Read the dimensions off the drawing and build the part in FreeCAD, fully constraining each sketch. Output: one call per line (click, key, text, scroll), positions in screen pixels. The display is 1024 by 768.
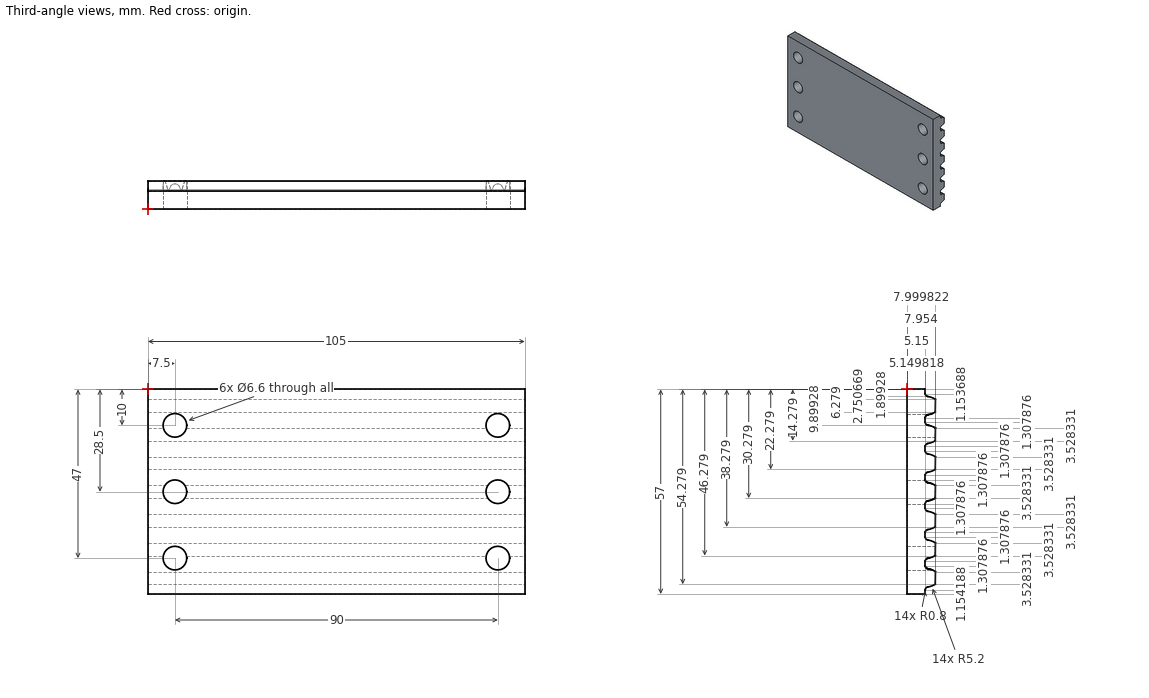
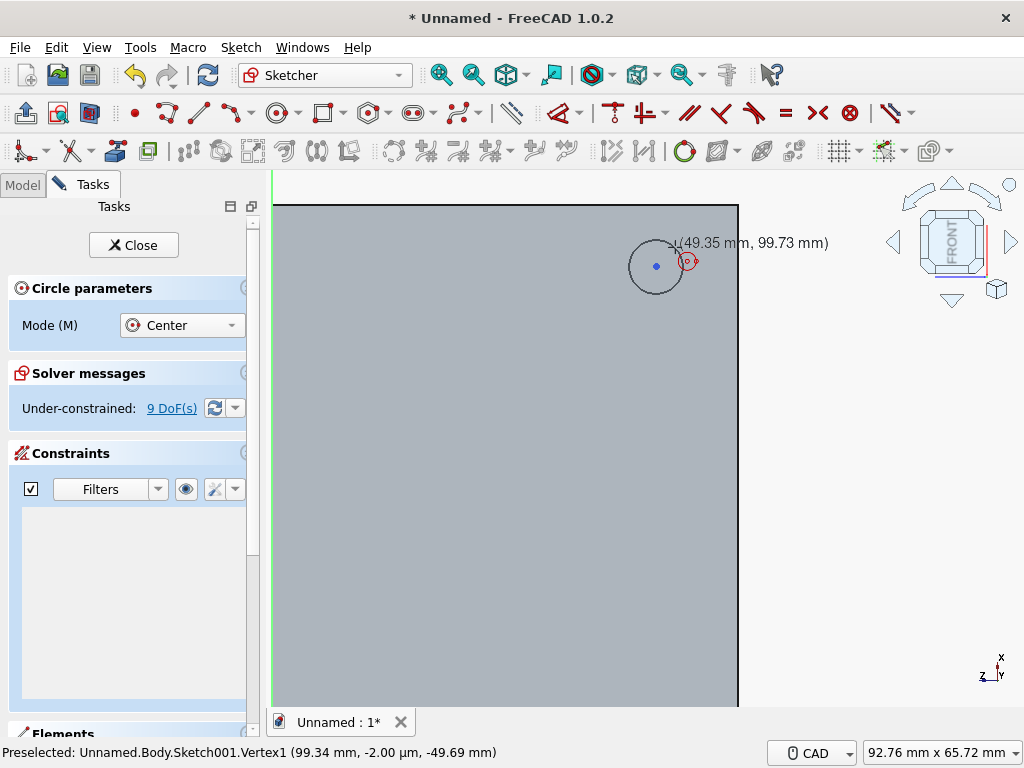
click(353, 266)
click(373, 247)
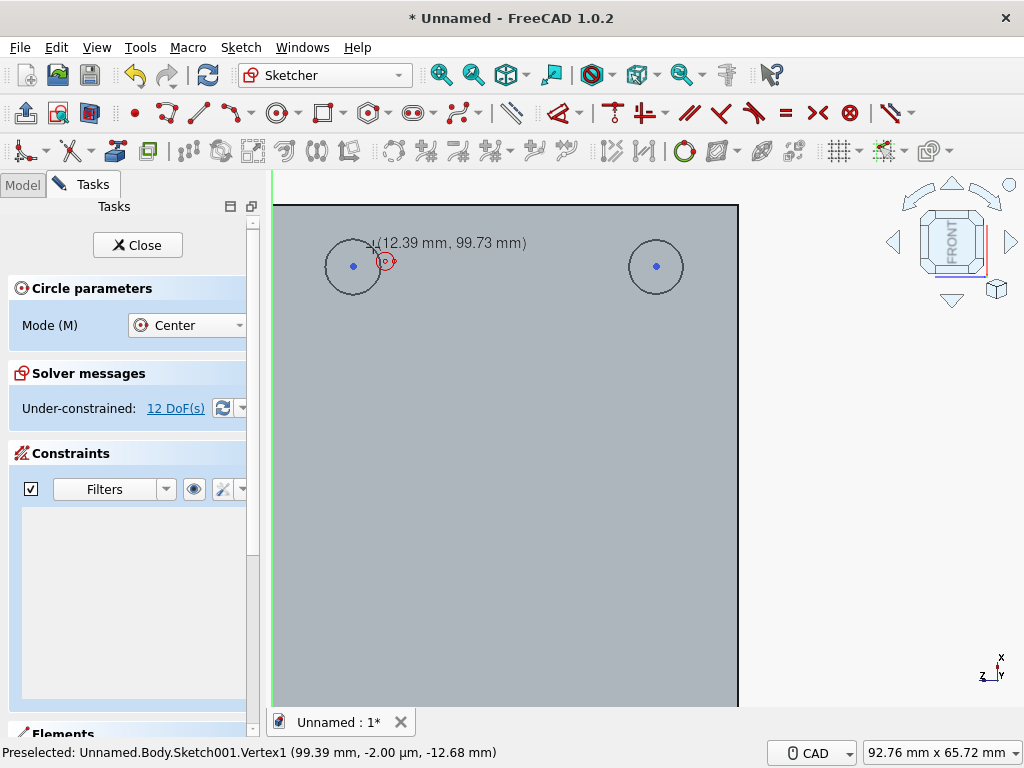
click(505, 266)
click(524, 247)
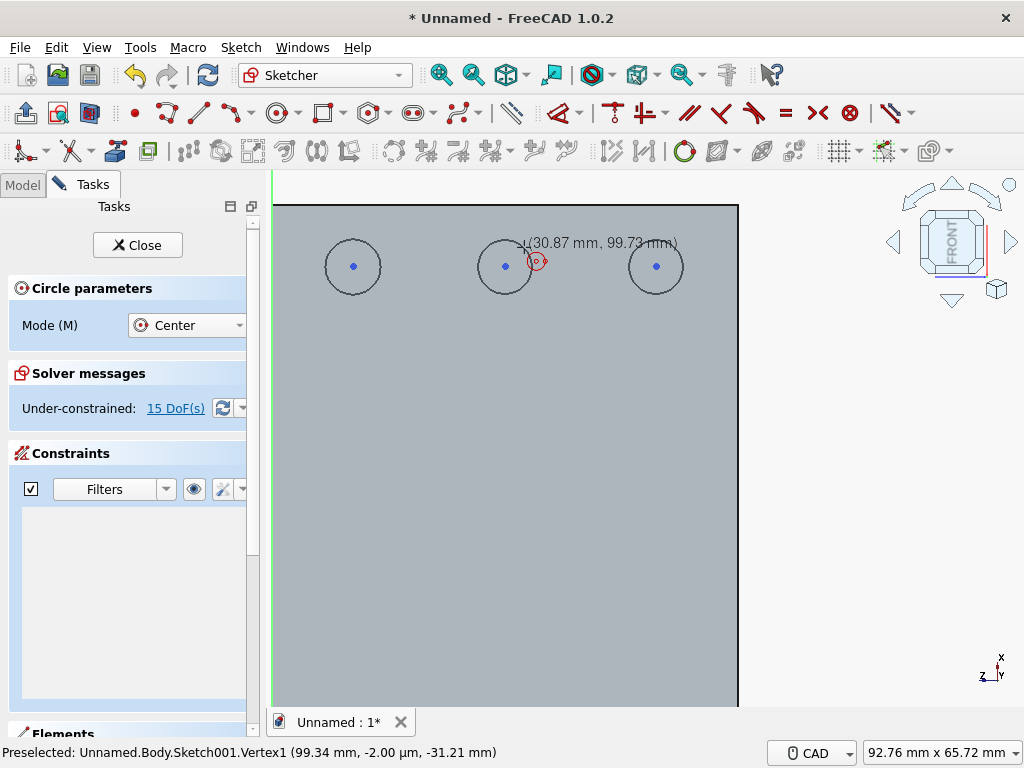
scroll(657, 265, down, 4)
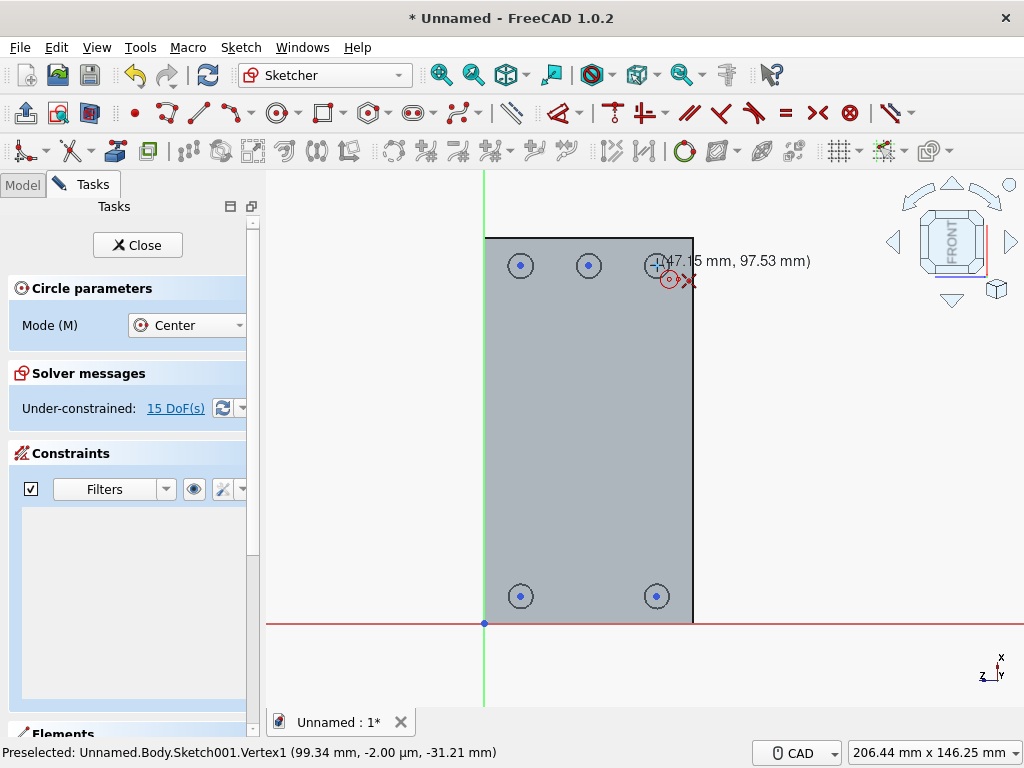
scroll(589, 596, up, 4)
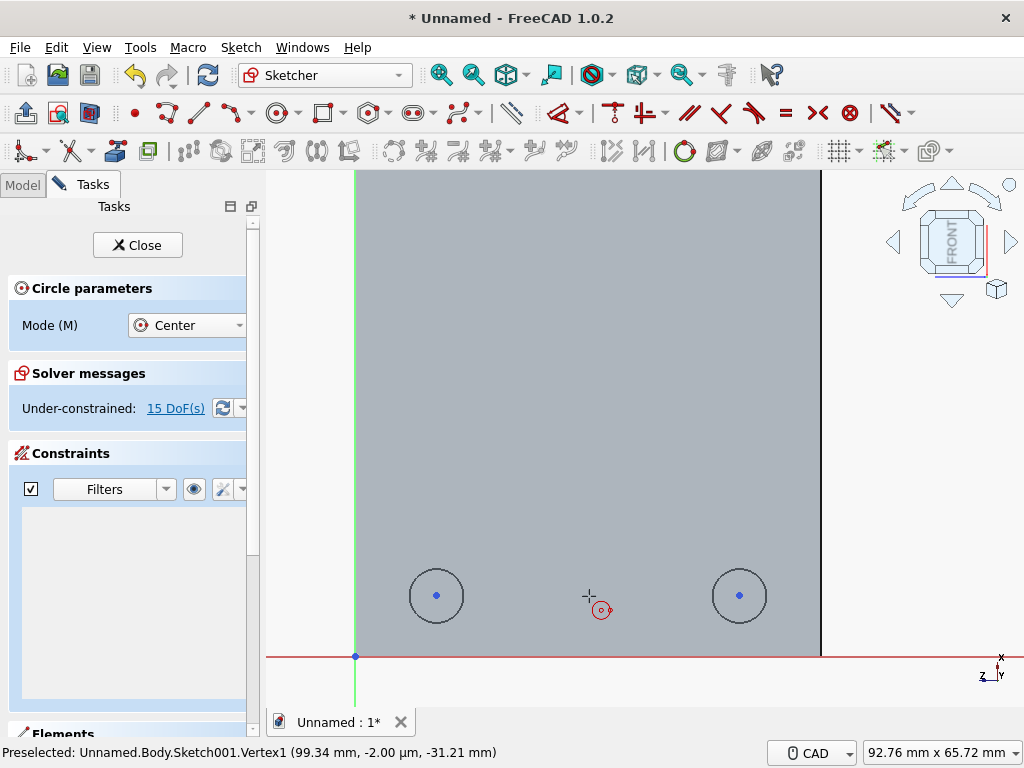
click(588, 595)
click(607, 576)
key(Escape)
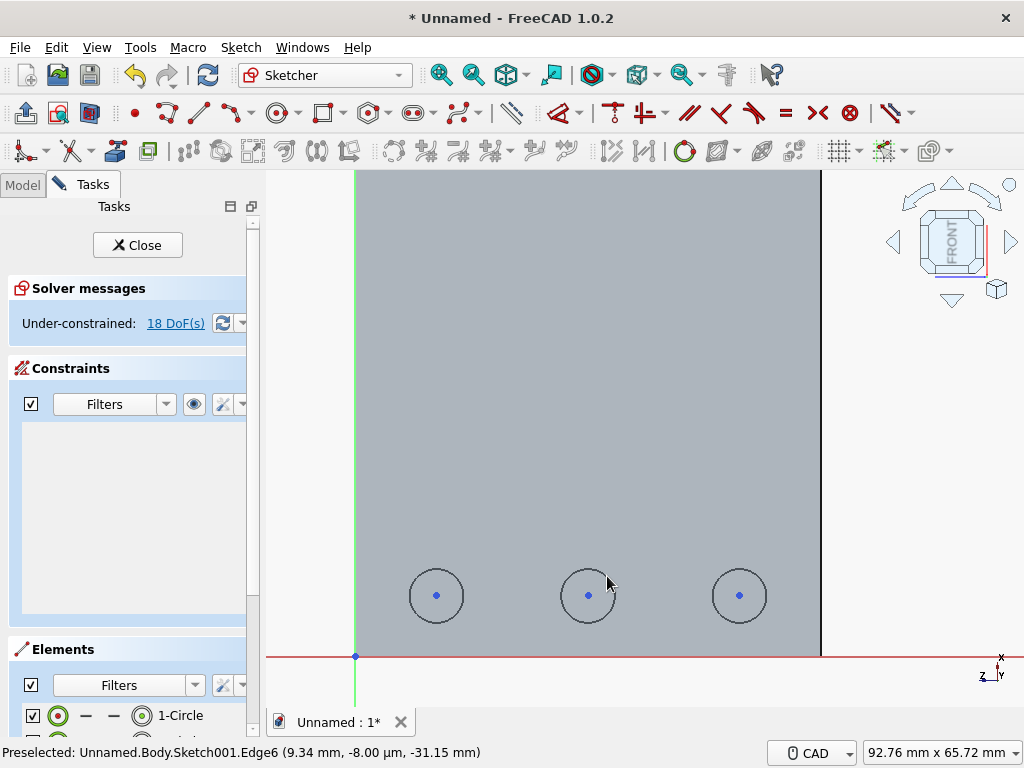
click(455, 577)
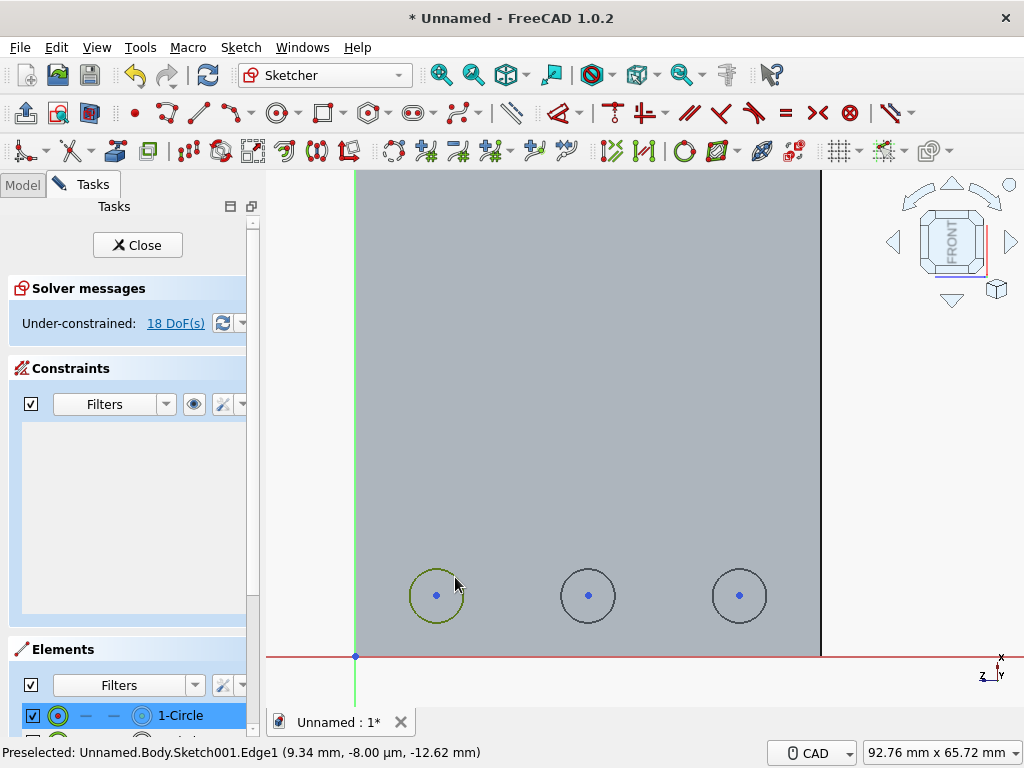
click(758, 577)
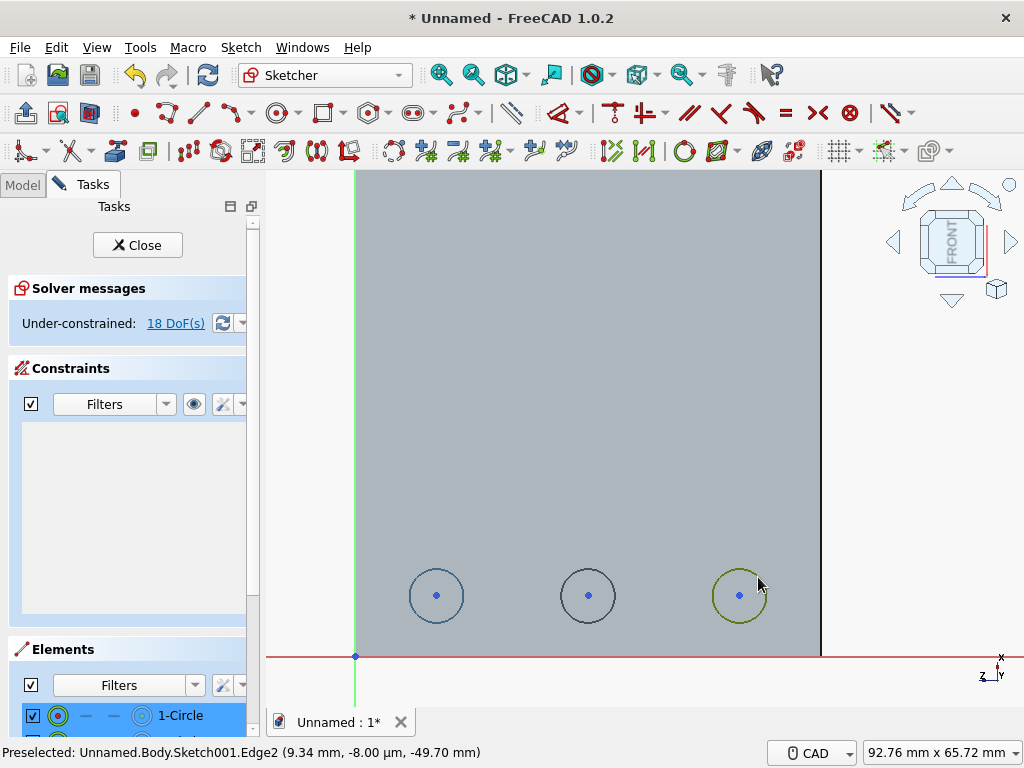
scroll(589, 597, down, 4)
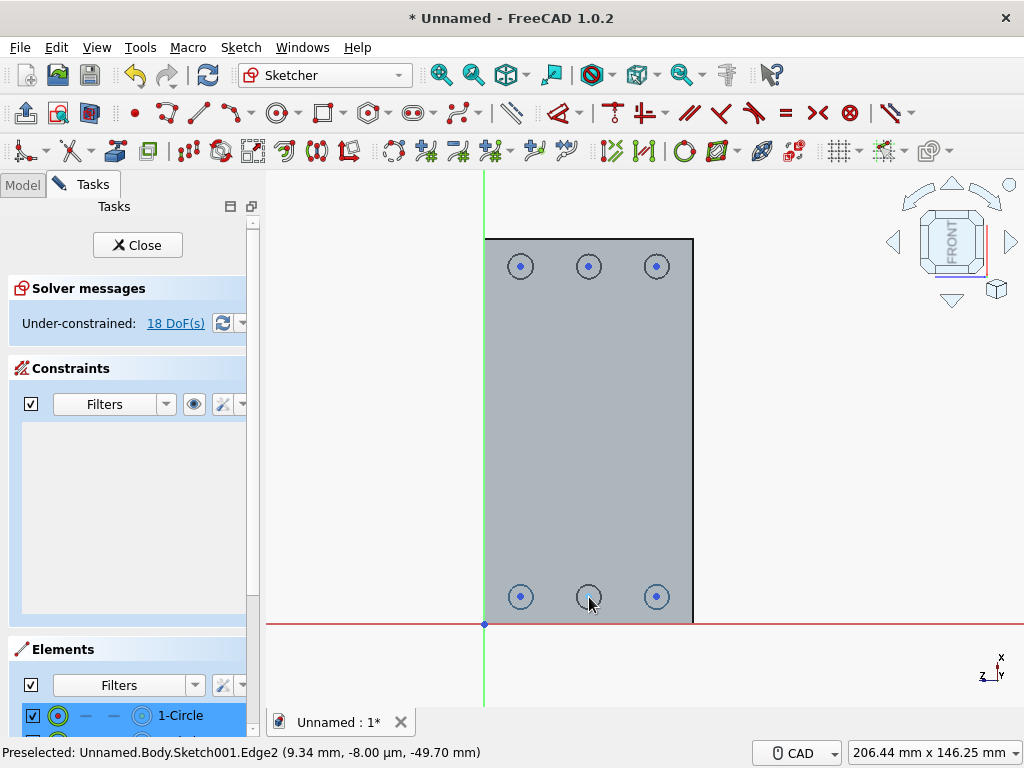
click(665, 258)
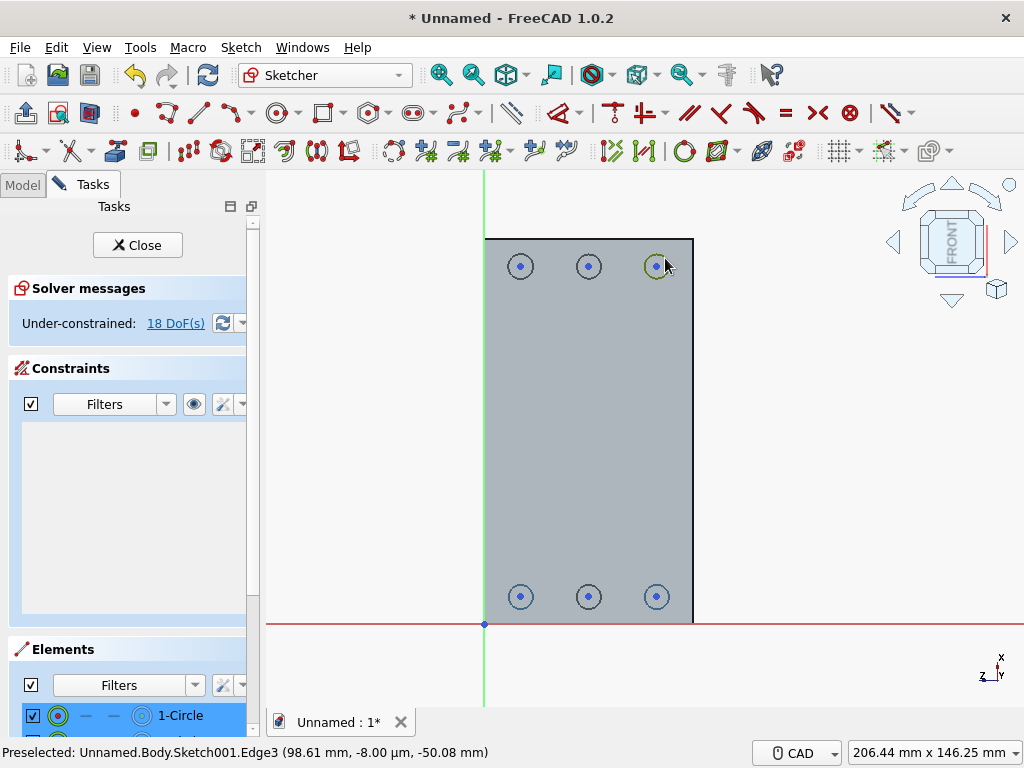
click(529, 258)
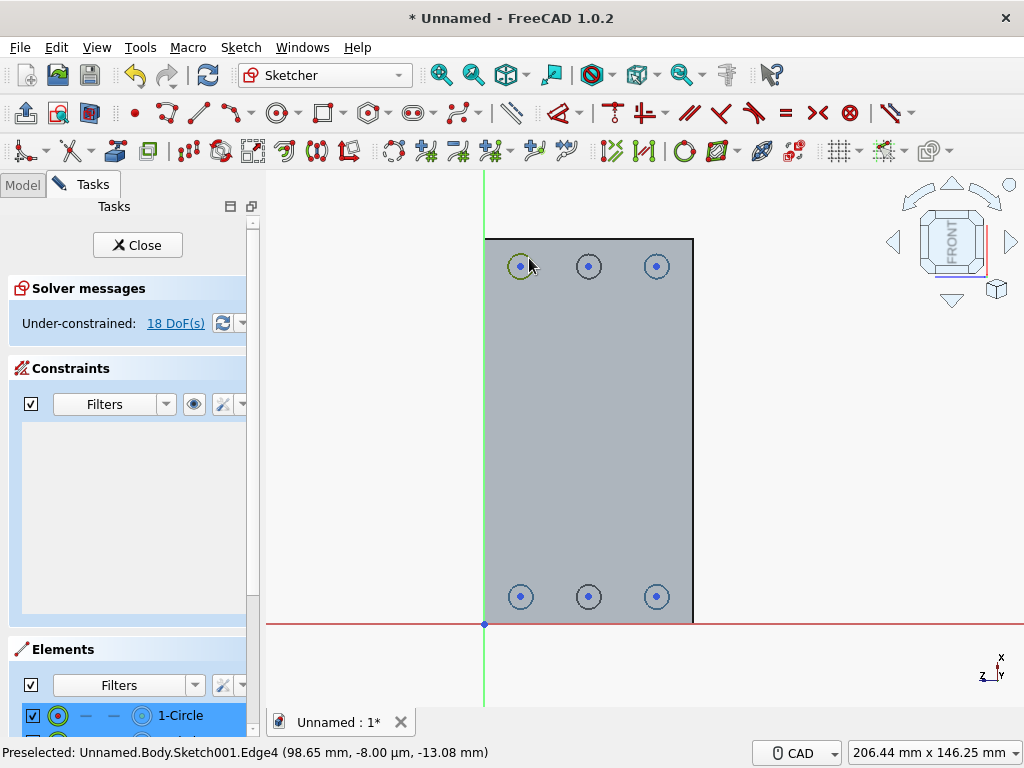
click(597, 258)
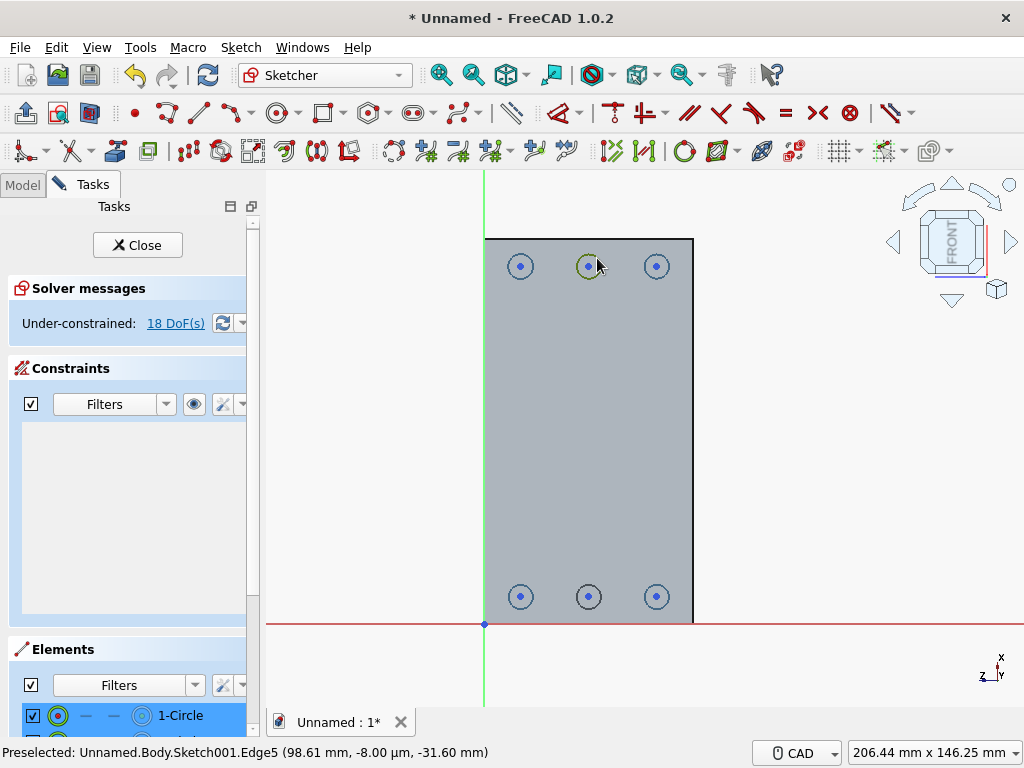
click(597, 588)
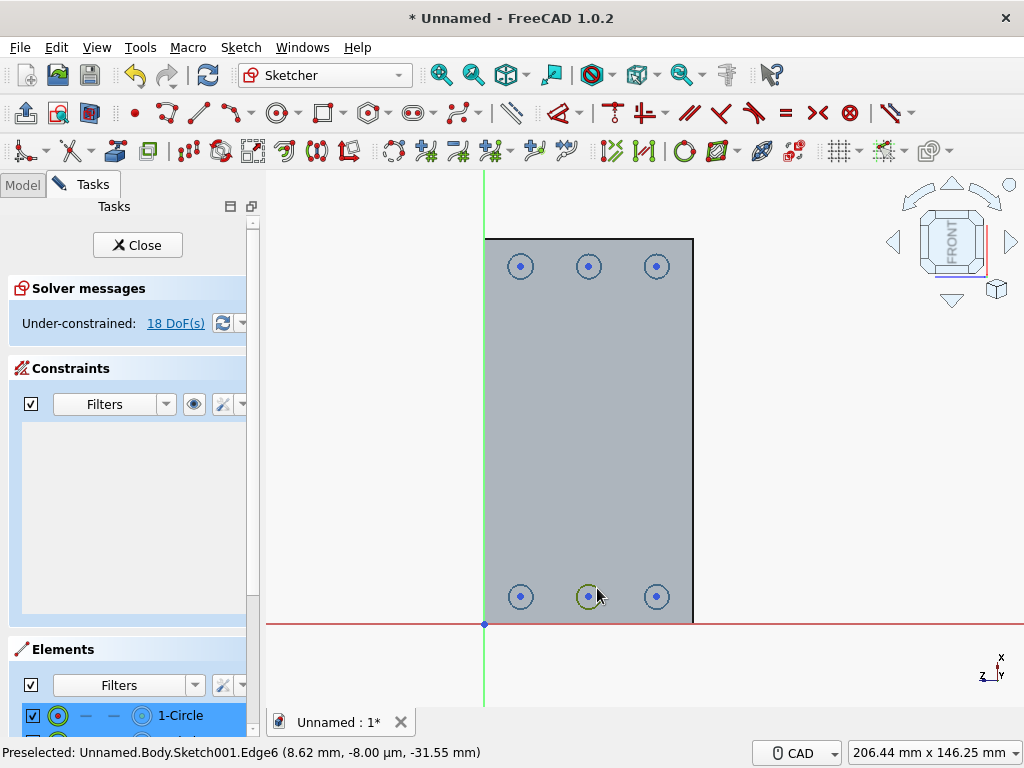
click(786, 114)